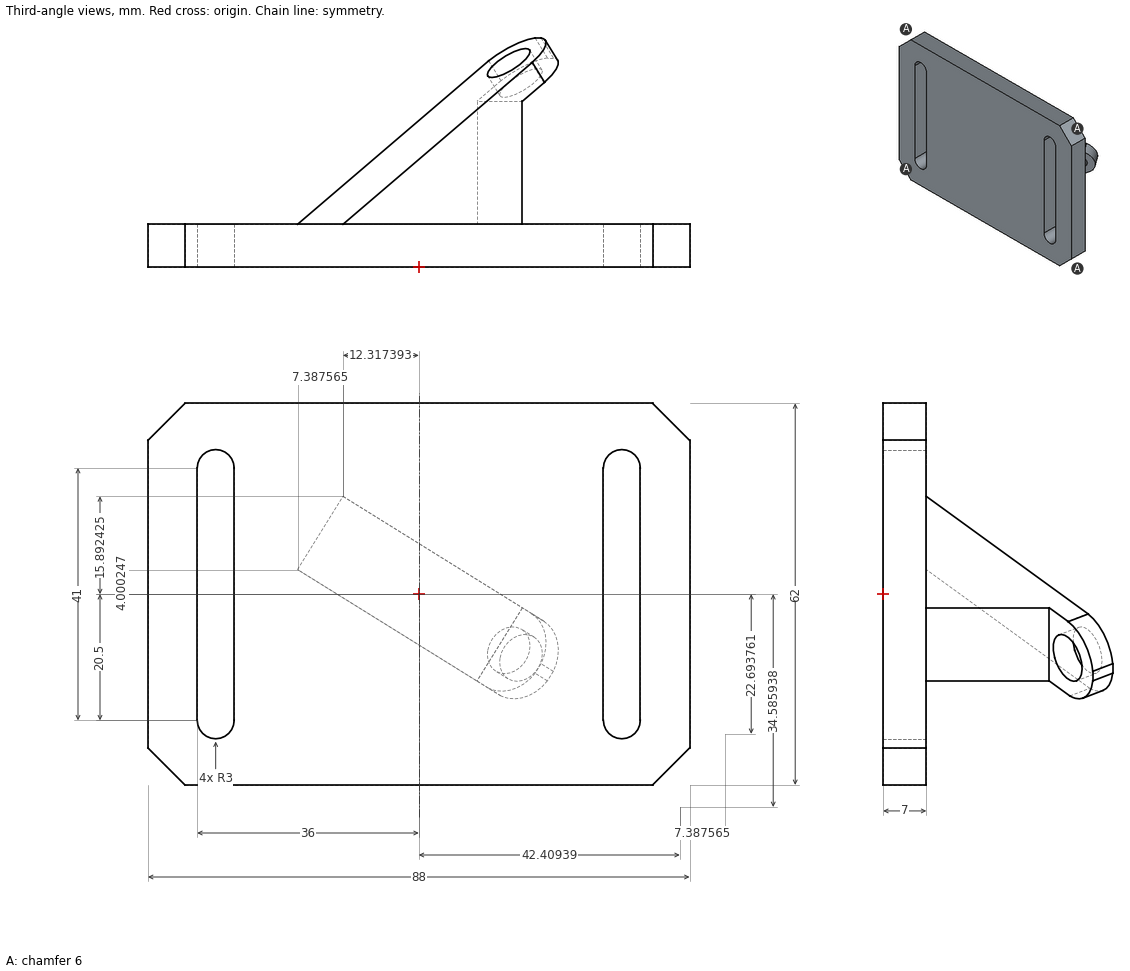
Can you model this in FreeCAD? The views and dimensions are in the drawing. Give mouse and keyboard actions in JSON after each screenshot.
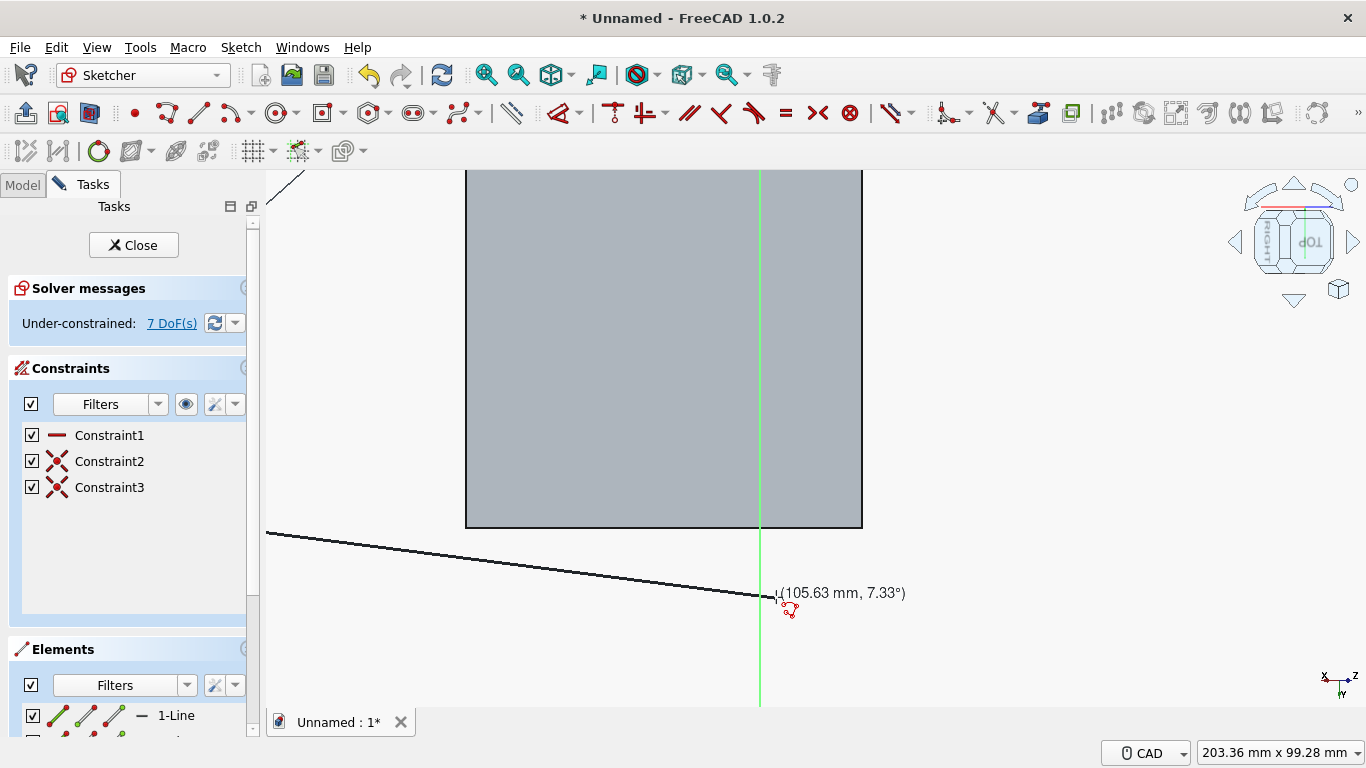
{"action": "left_click", "coordinate": [776, 596]}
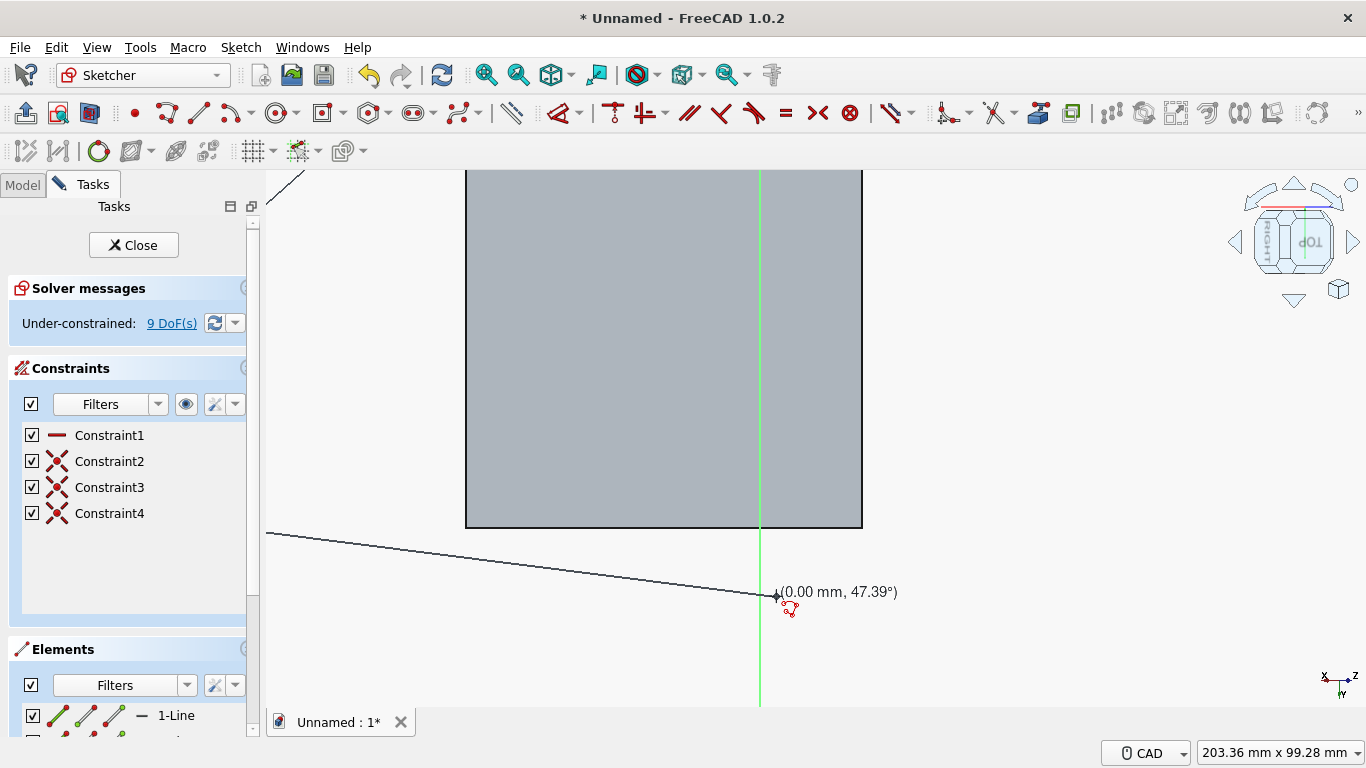
{"action": "scroll", "coordinate": [776, 597], "scroll_direction": "down", "scroll_amount": 3}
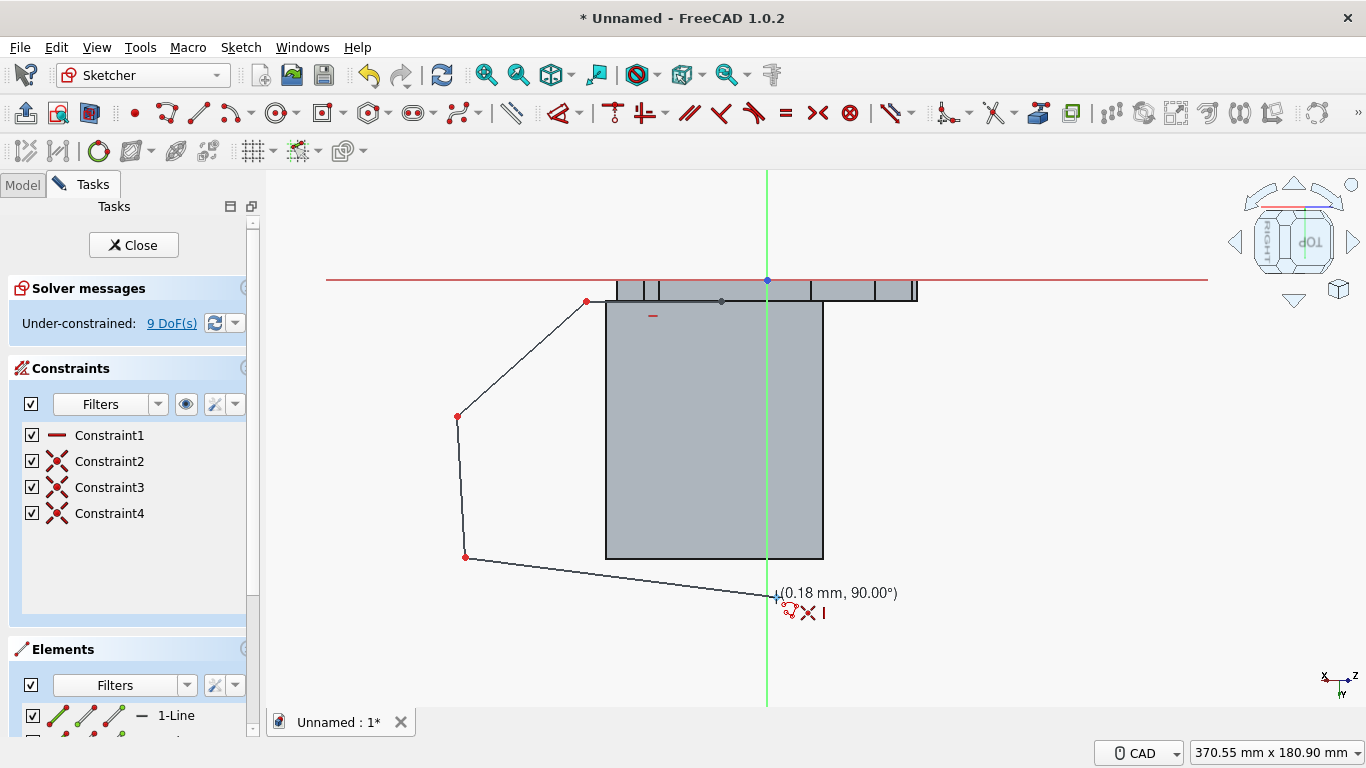
{"action": "left_click", "coordinate": [1038, 542]}
{"action": "left_click", "coordinate": [823, 301]}
{"action": "left_click", "coordinate": [699, 391]}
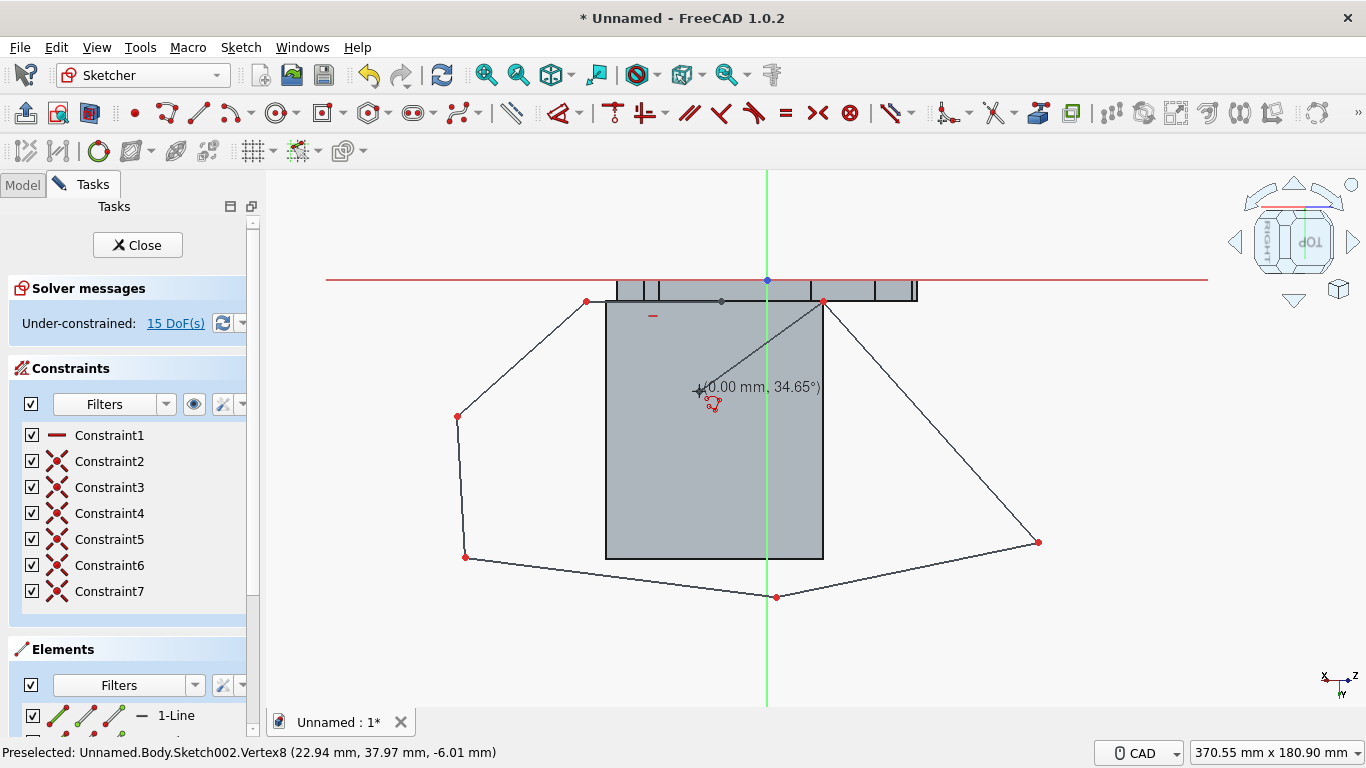
{"action": "scroll", "coordinate": [692, 381], "scroll_direction": "up", "scroll_amount": 2}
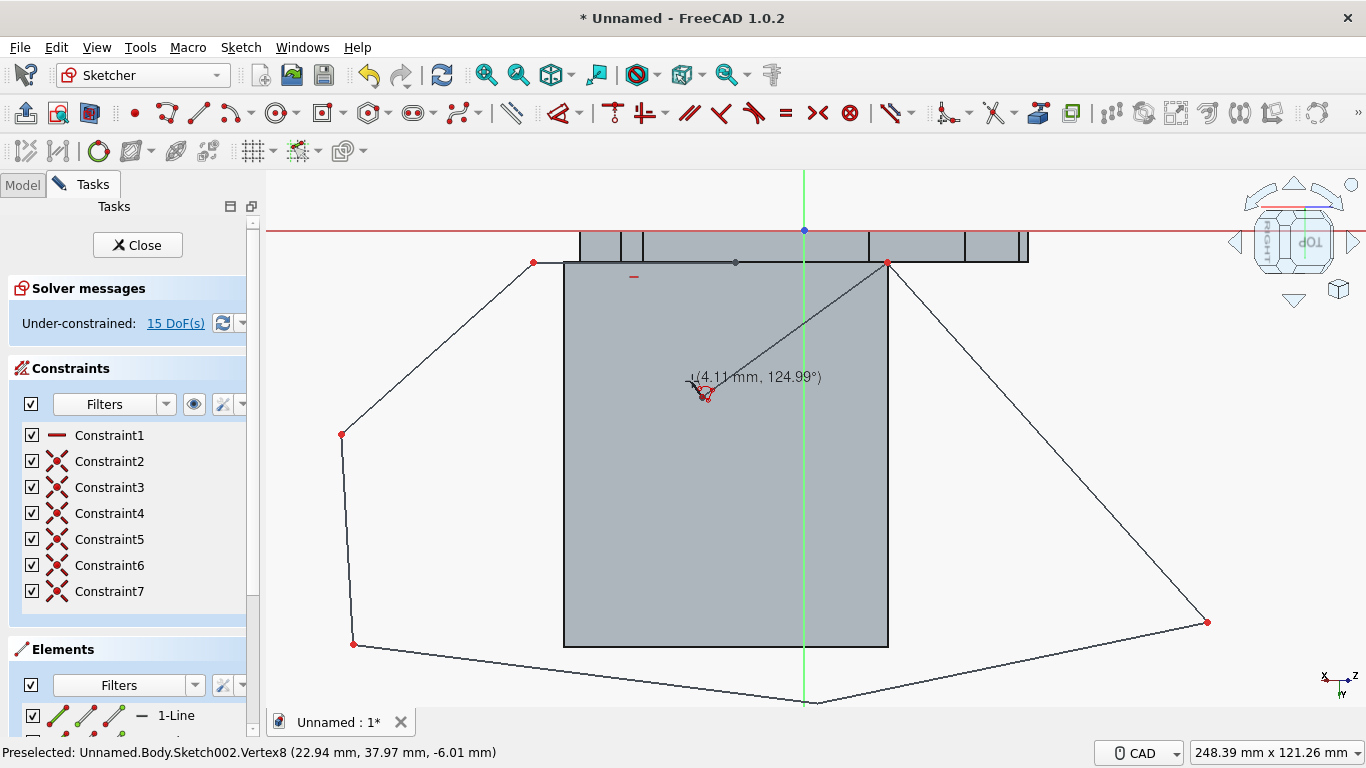
{"action": "left_click", "coordinate": [692, 381]}
{"action": "left_click", "coordinate": [735, 350]}
{"action": "left_click", "coordinate": [735, 263]}
{"action": "key", "text": "Escape"}
{"action": "key", "text": "Escape"}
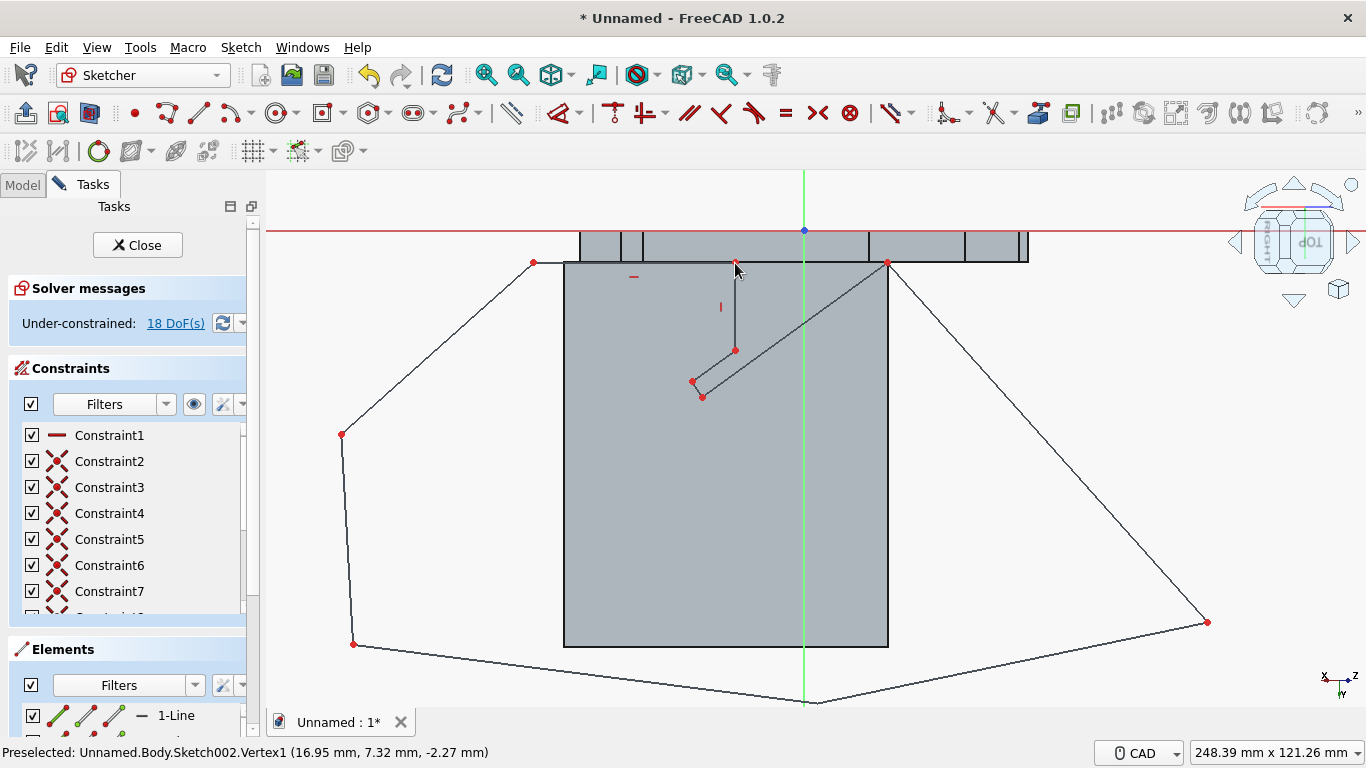
{"action": "left_click", "coordinate": [558, 114]}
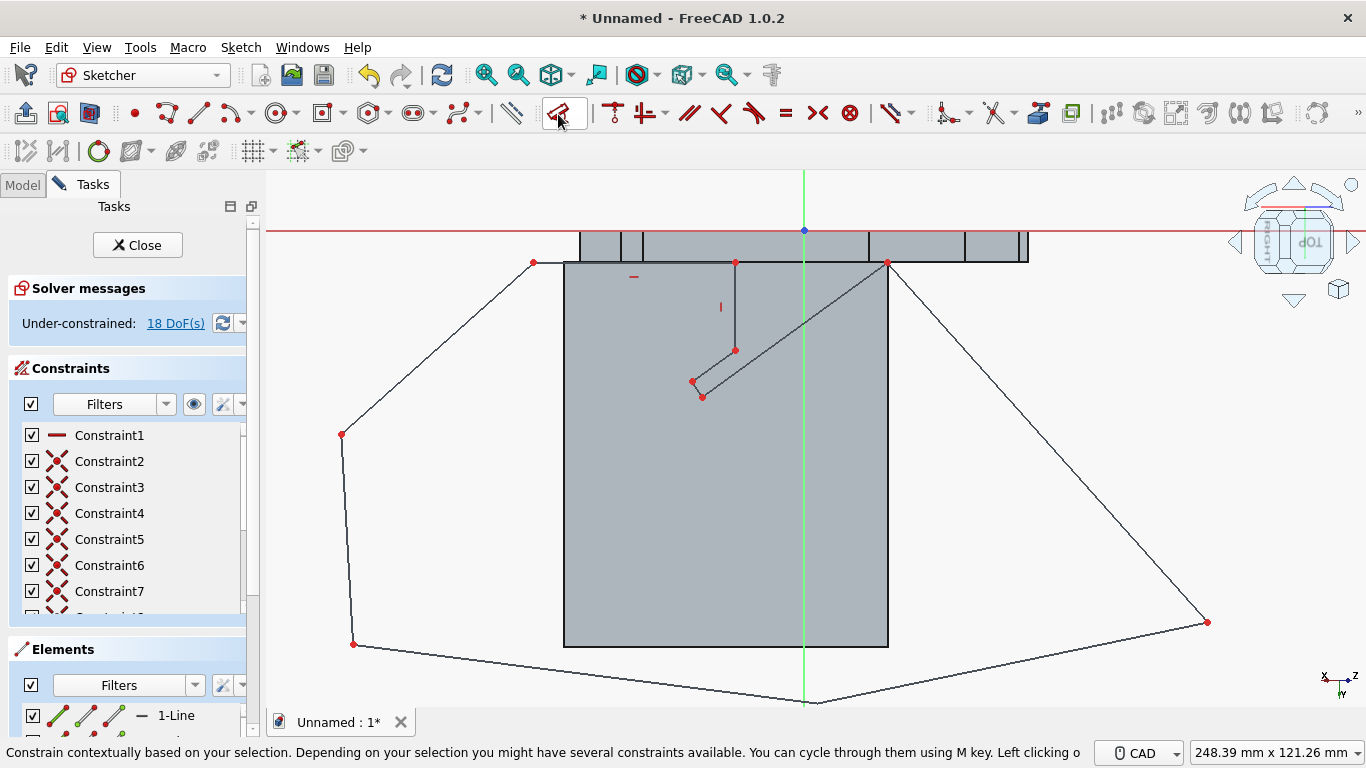
{"action": "left_click", "coordinate": [735, 325]}
{"action": "left_click", "coordinate": [701, 307]}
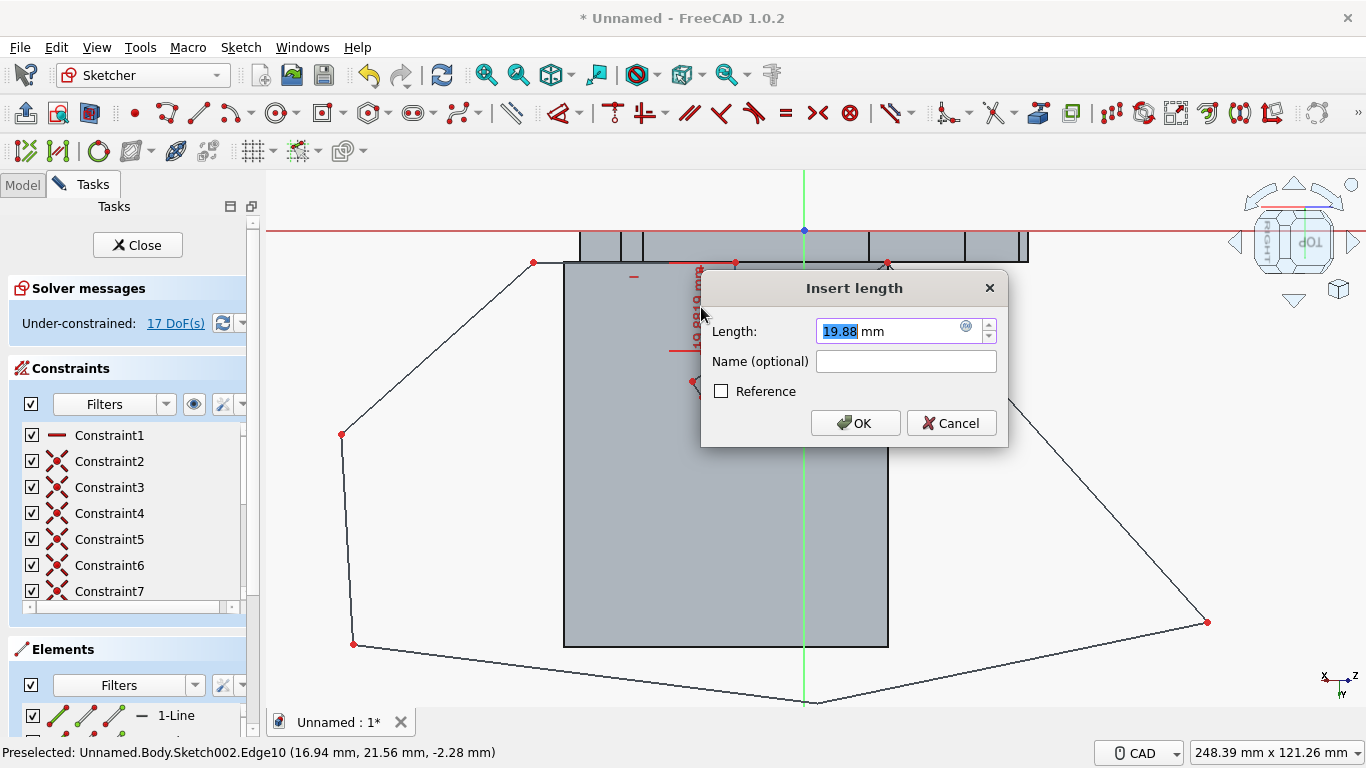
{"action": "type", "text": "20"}
{"action": "key", "text": "Return"}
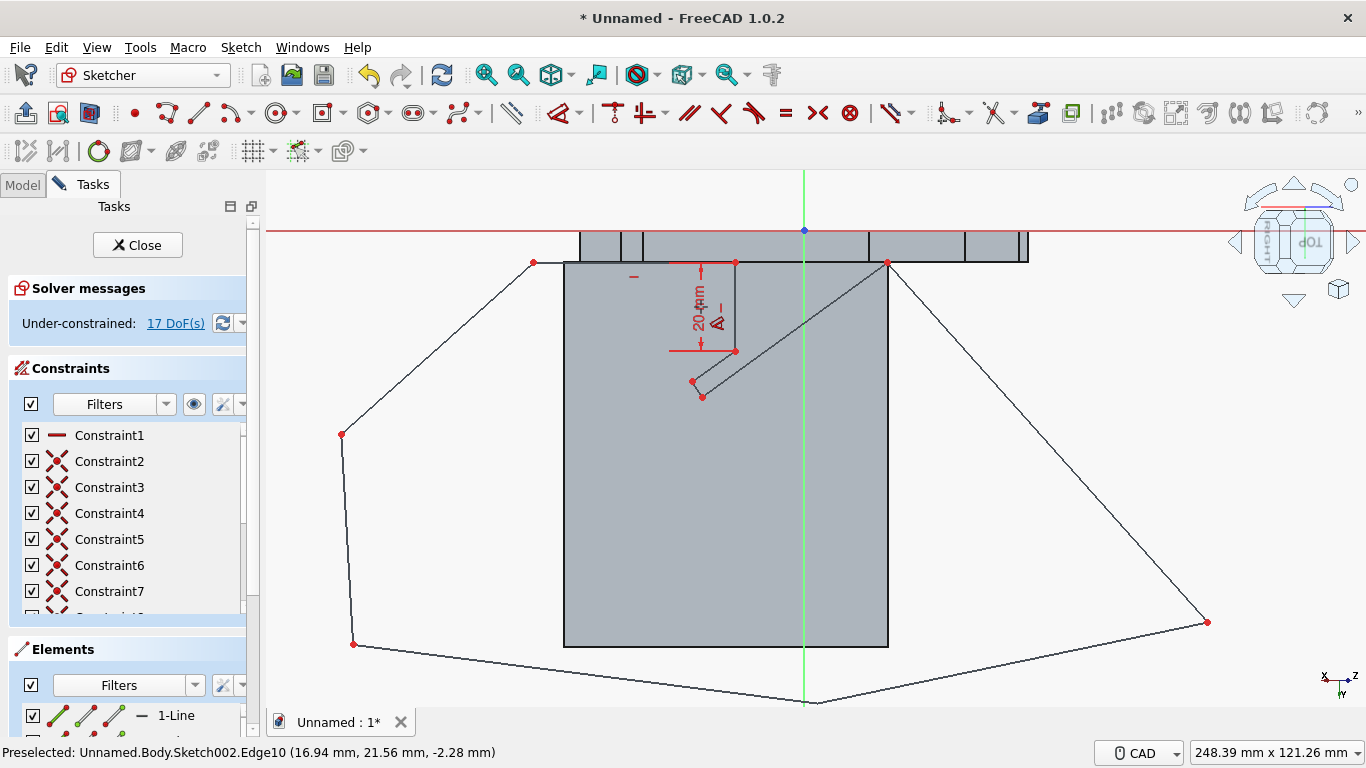
{"action": "scroll", "coordinate": [735, 263], "scroll_direction": "up", "scroll_amount": 2}